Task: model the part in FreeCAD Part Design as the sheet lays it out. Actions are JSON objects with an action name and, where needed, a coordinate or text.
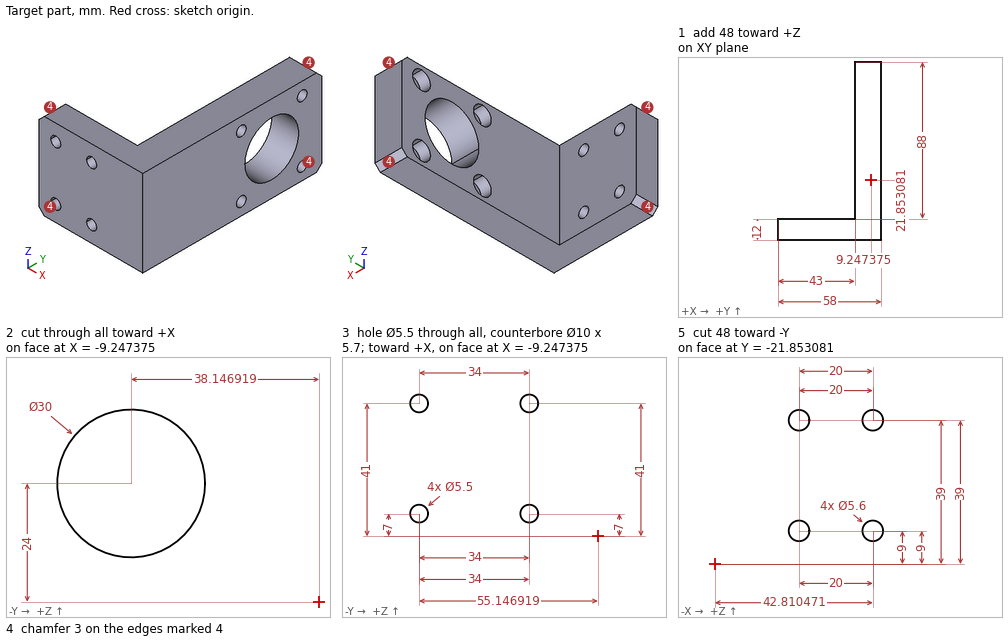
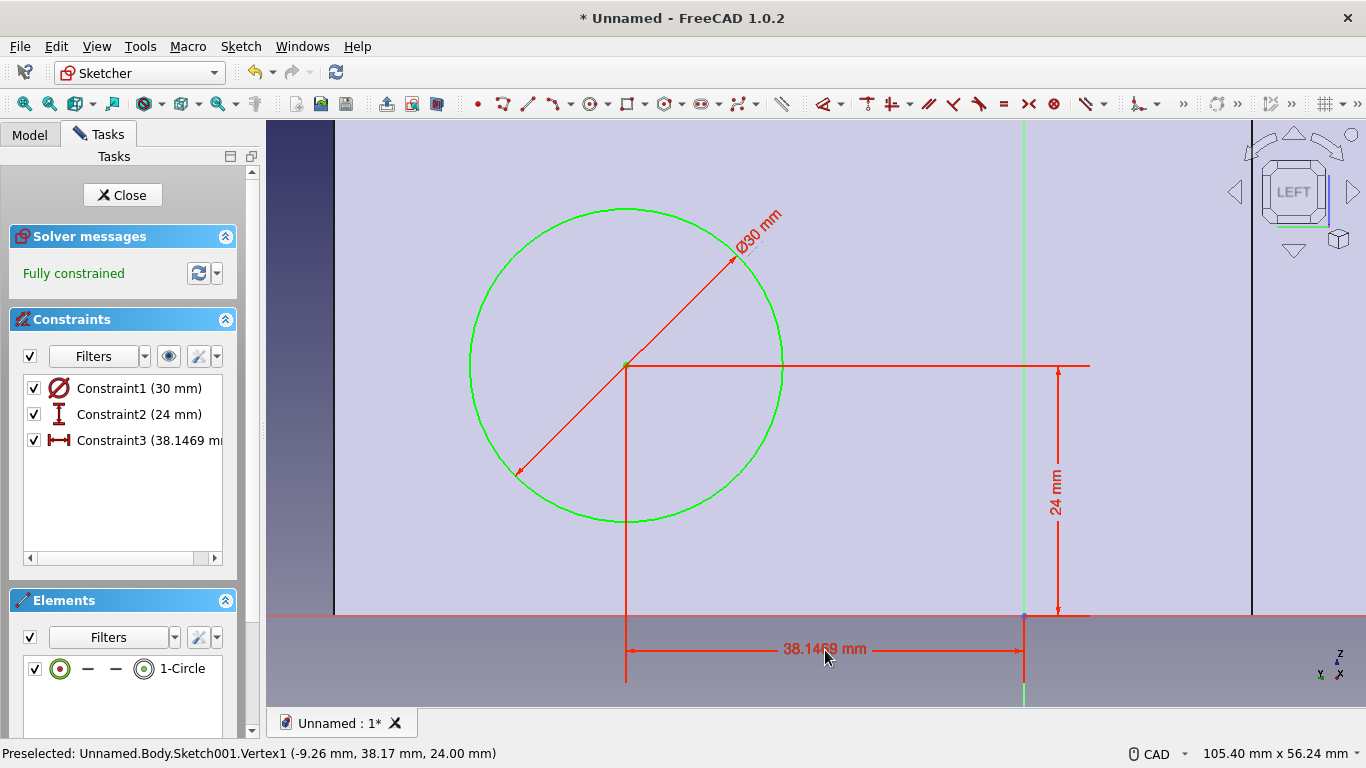
{"action": "left_click", "coordinate": [123, 195]}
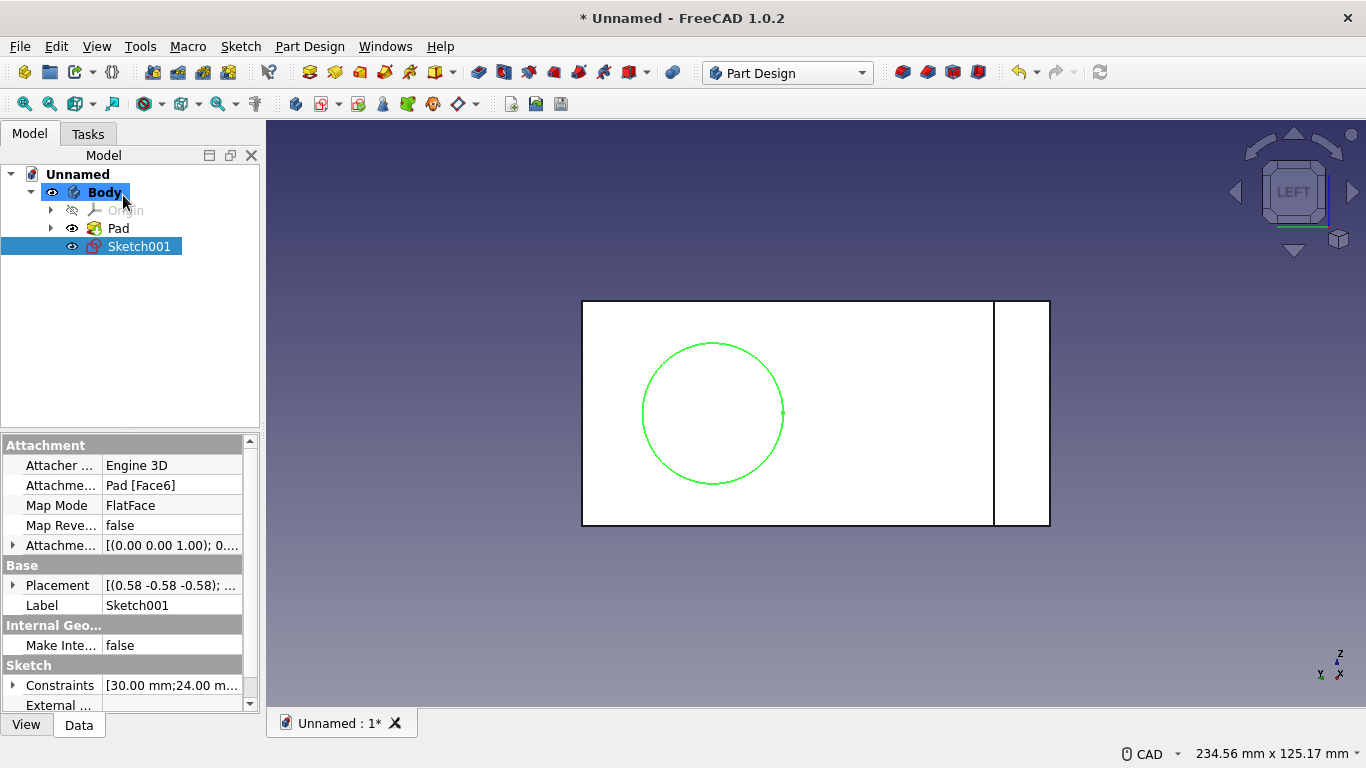
{"action": "left_click", "coordinate": [479, 72]}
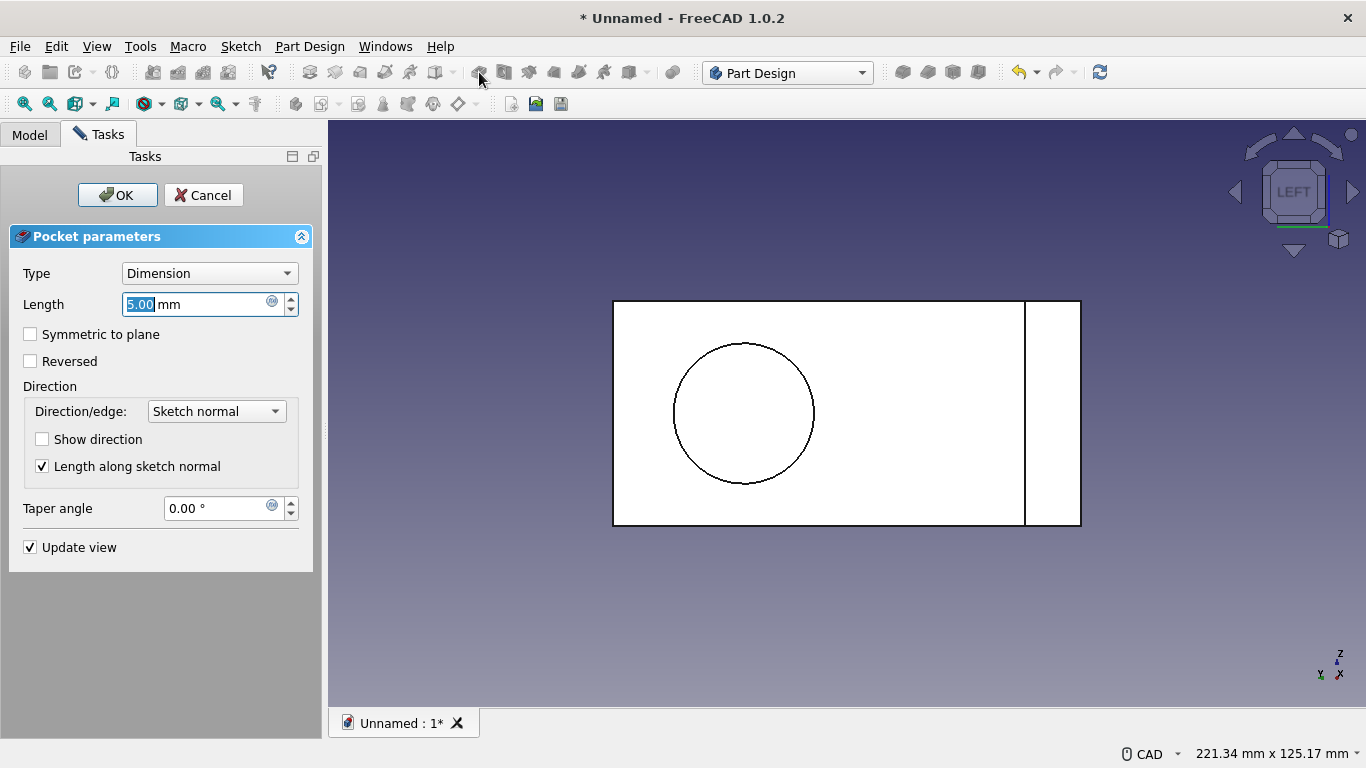
{"action": "left_click", "coordinate": [210, 274]}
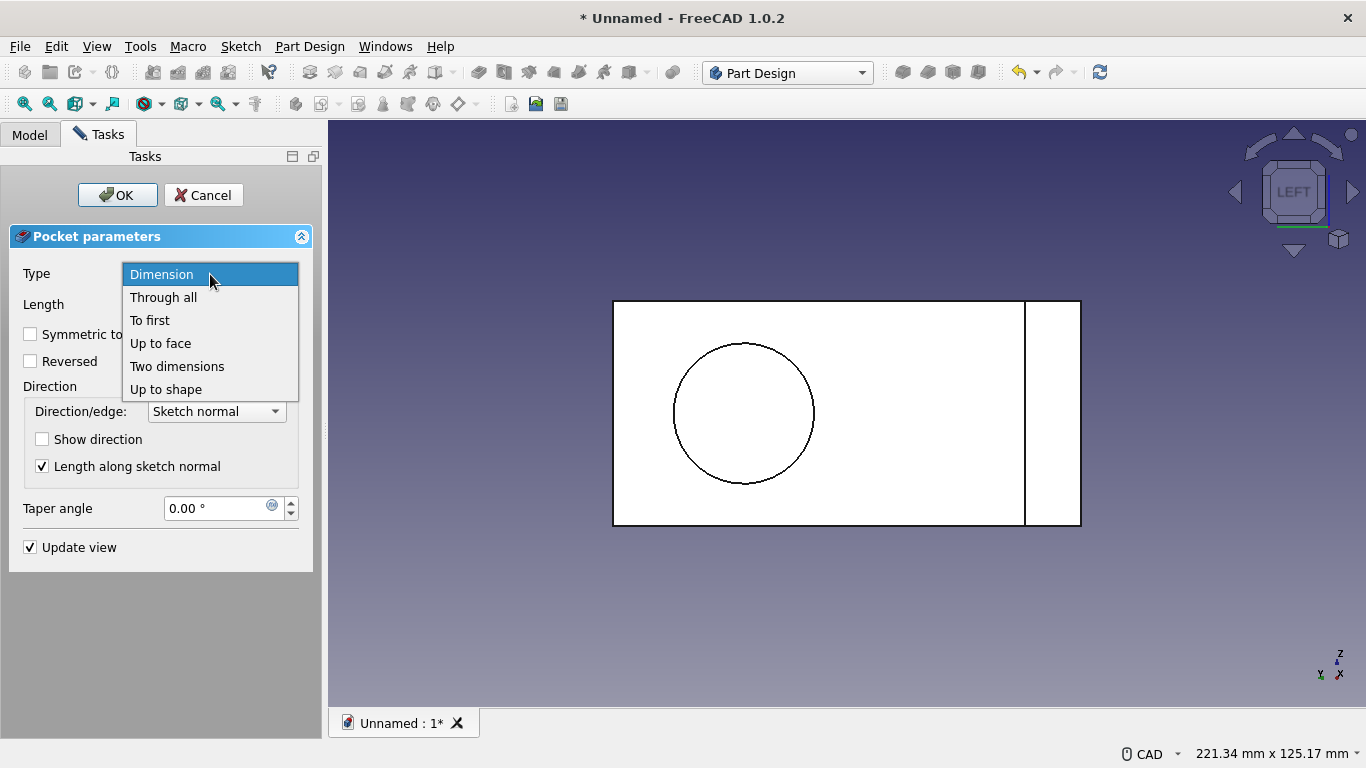
{"action": "left_click", "coordinate": [208, 298]}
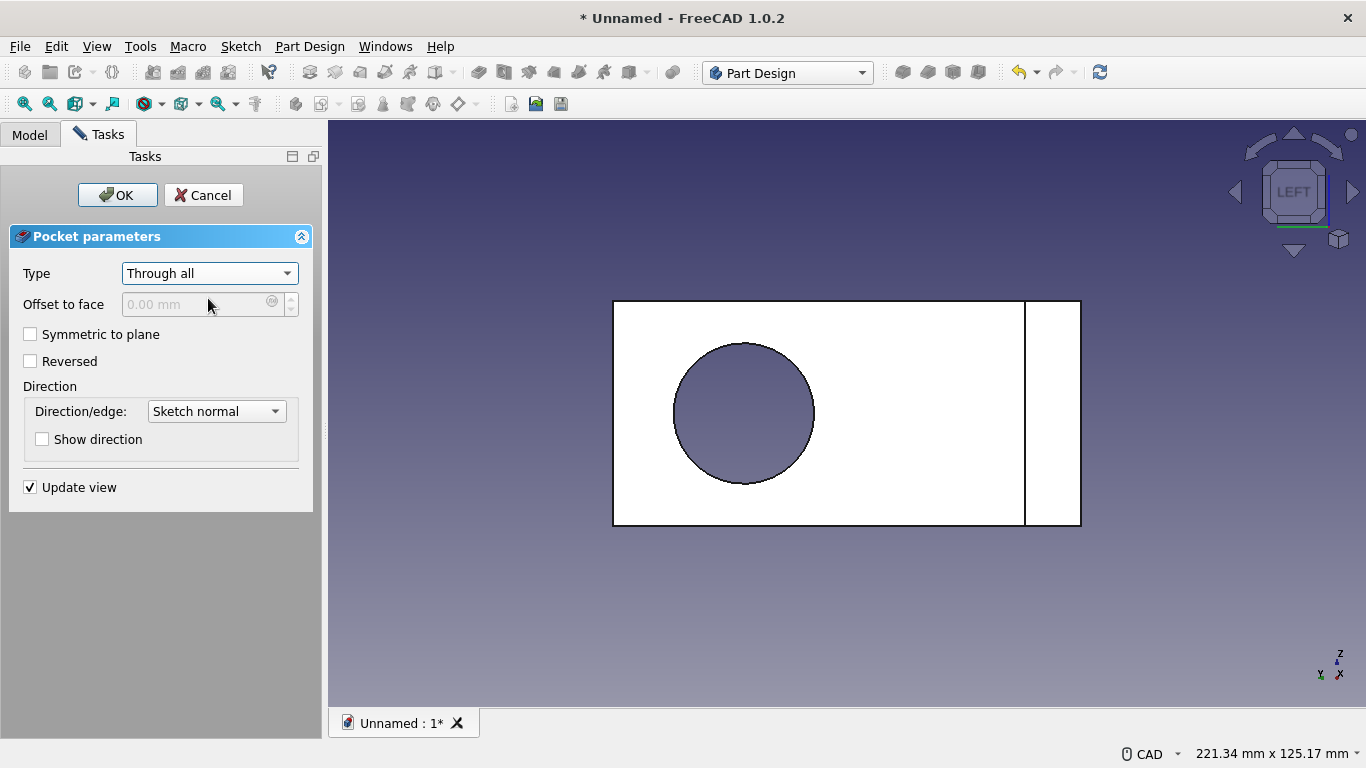
{"action": "left_click", "coordinate": [118, 195]}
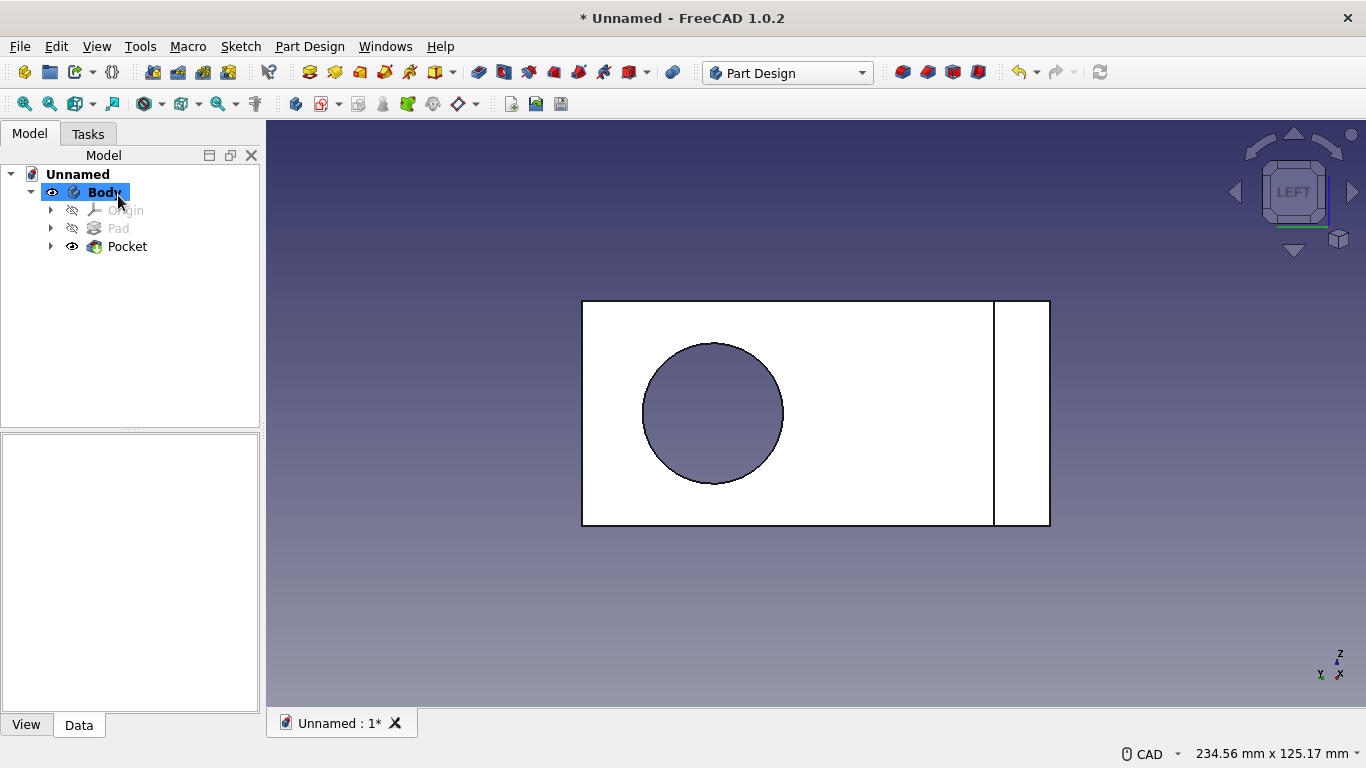
{"action": "left_click", "coordinate": [25, 104]}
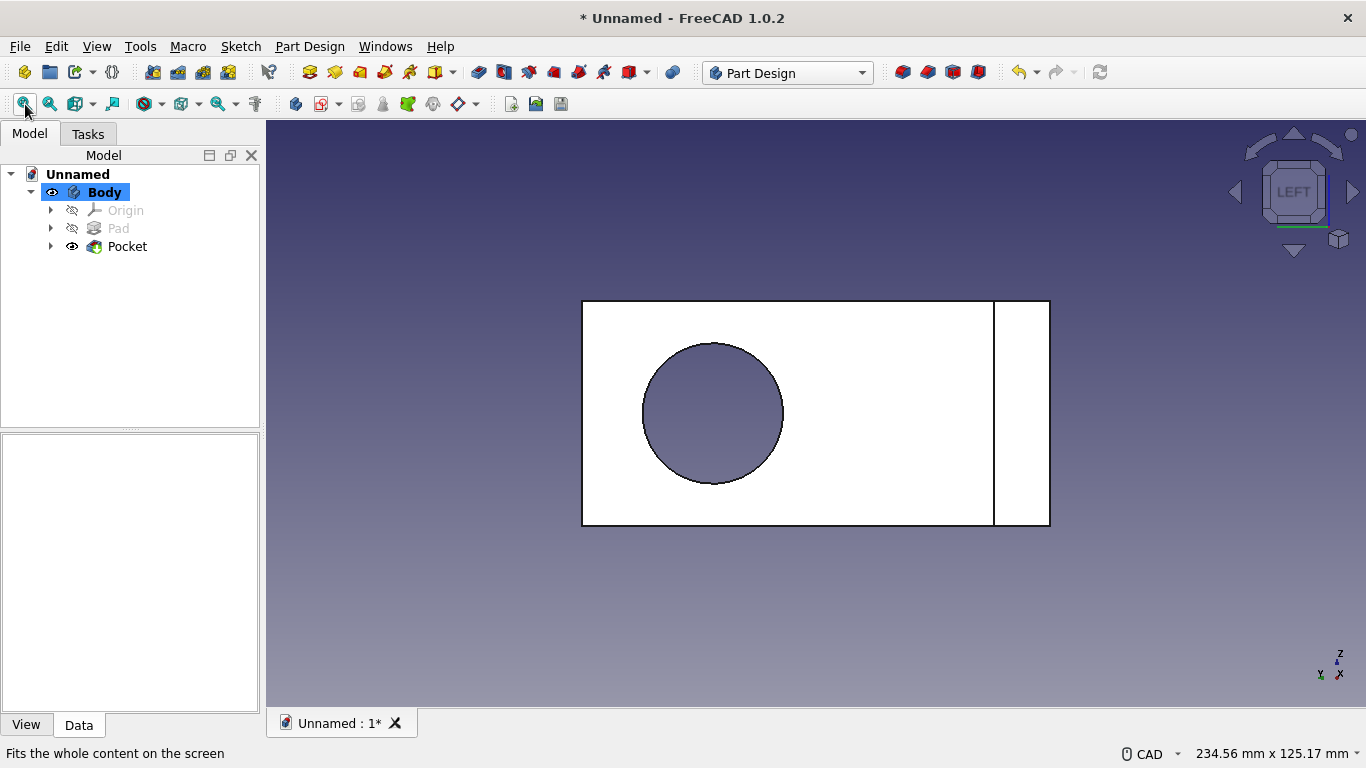
{"action": "left_click", "coordinate": [906, 412]}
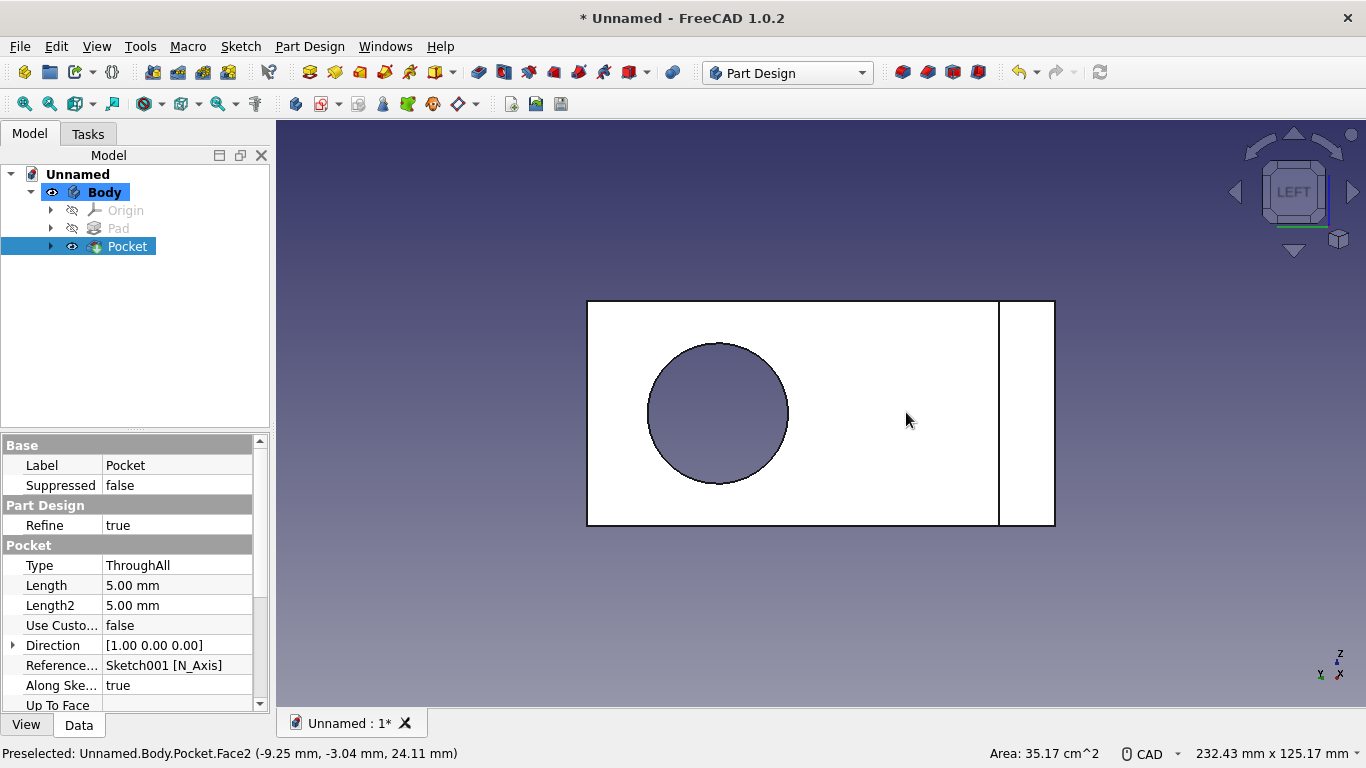
{"action": "left_click", "coordinate": [320, 104]}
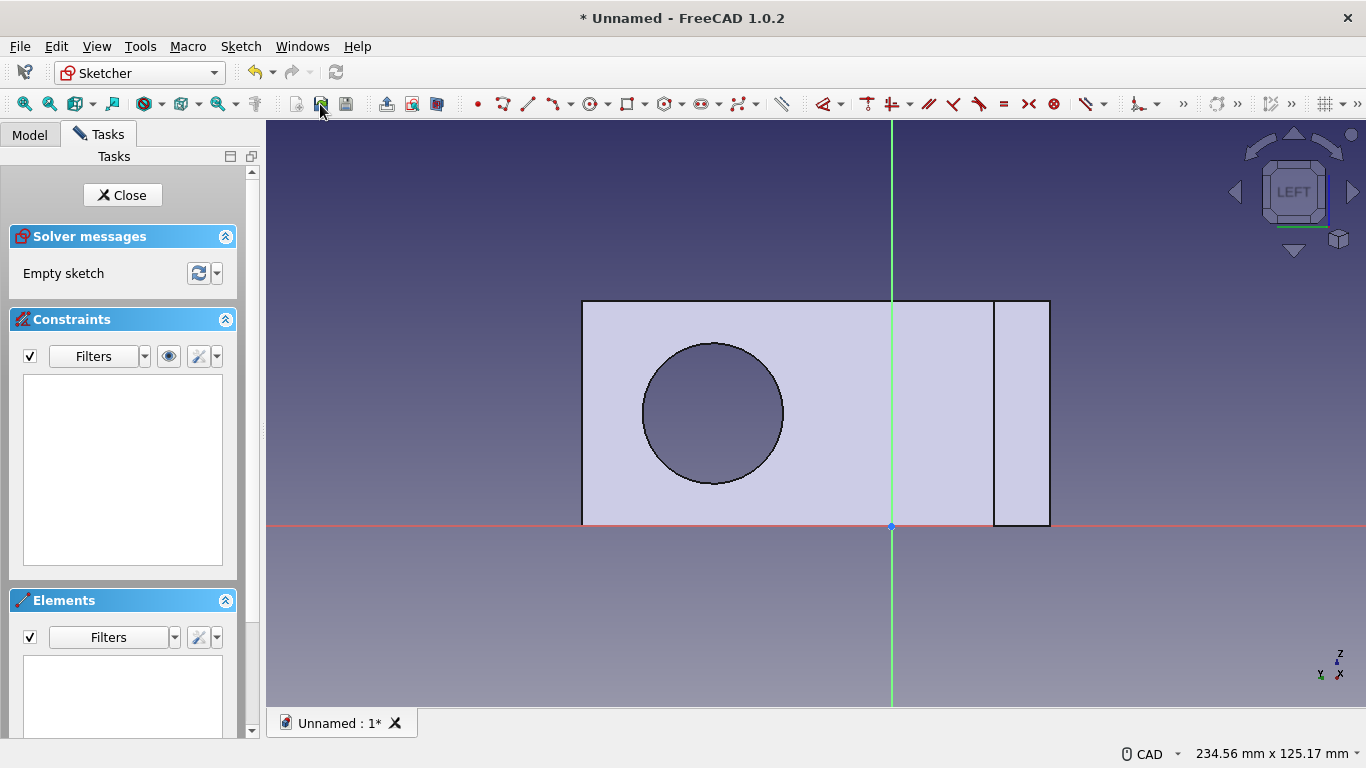
{"action": "key", "text": "q s"}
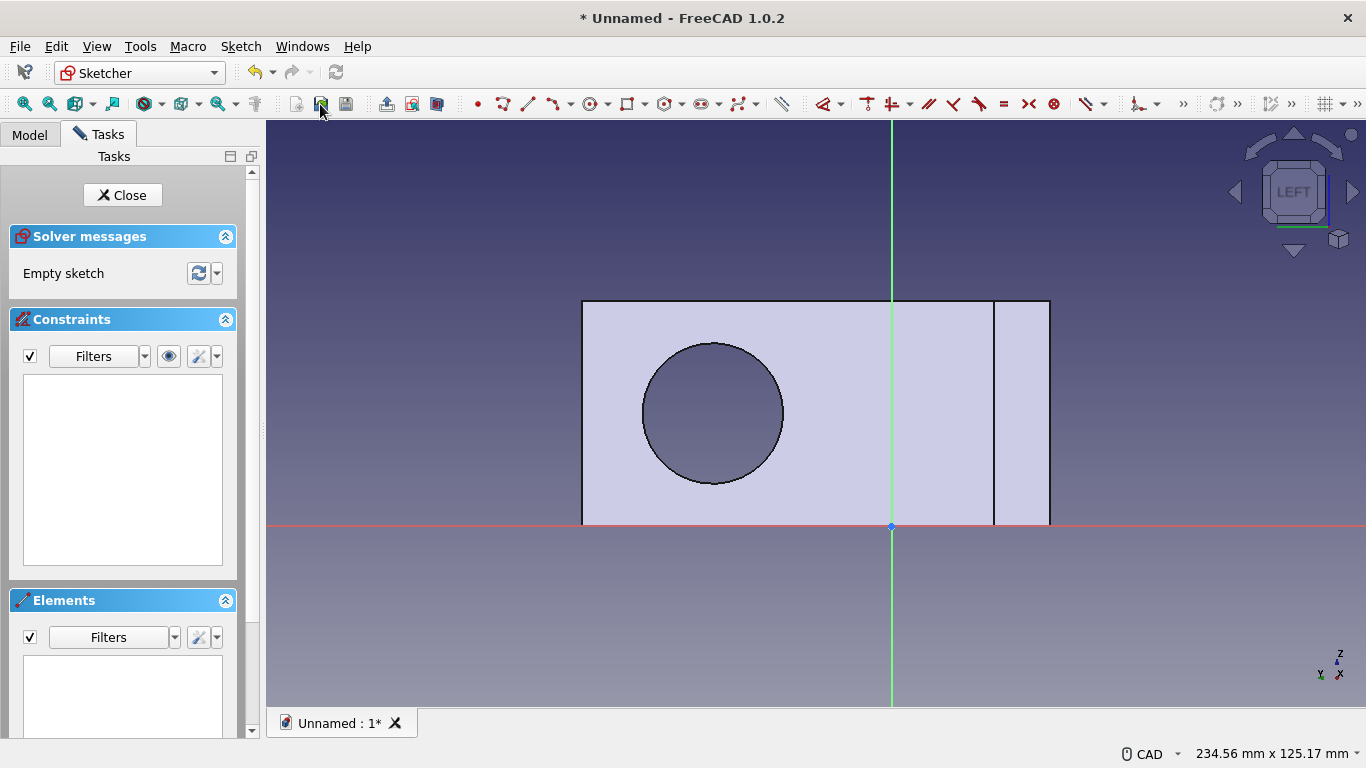
{"action": "scroll", "coordinate": [766, 436], "scroll_direction": "up", "scroll_amount": 3}